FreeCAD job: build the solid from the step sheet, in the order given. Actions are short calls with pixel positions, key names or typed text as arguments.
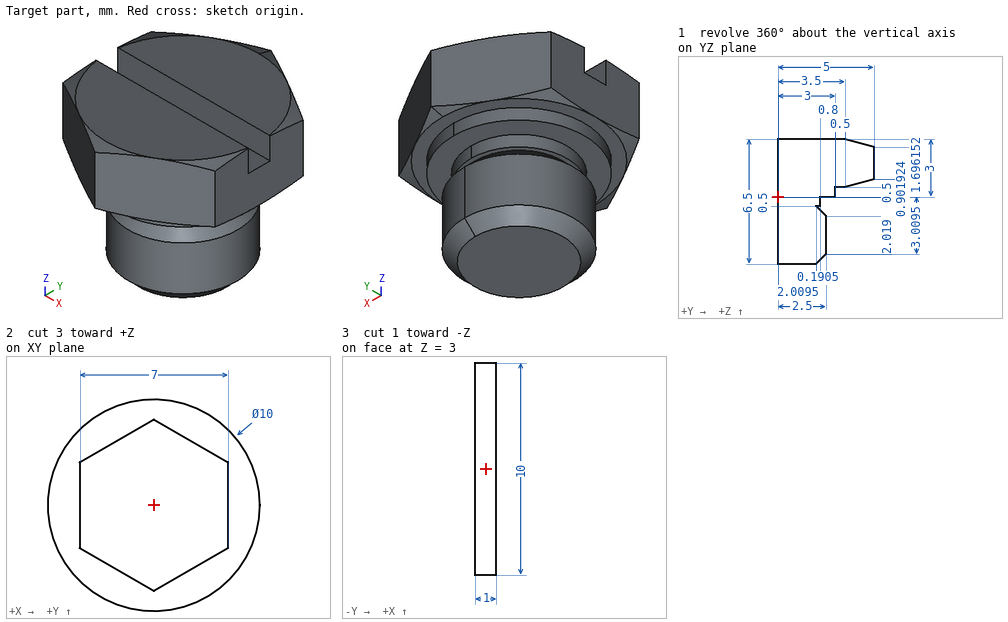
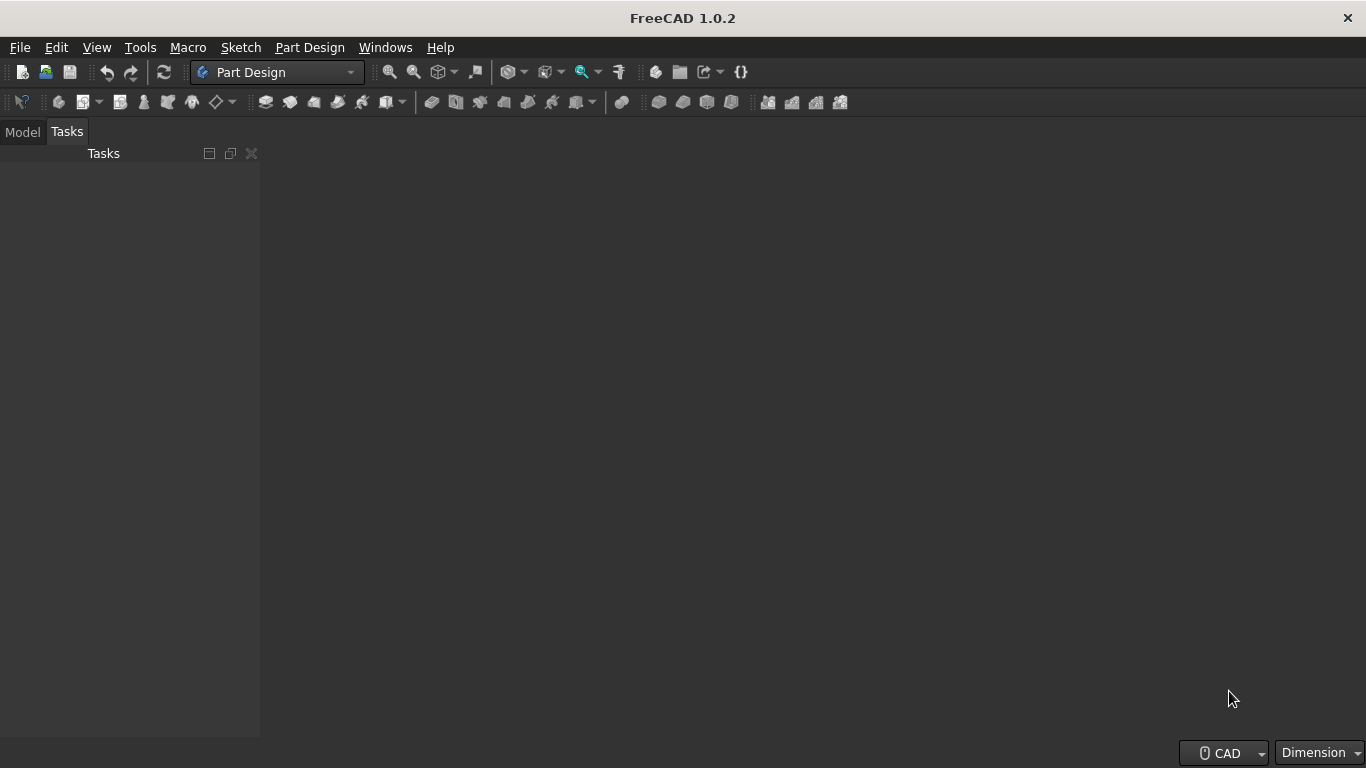
key(ctrl+n)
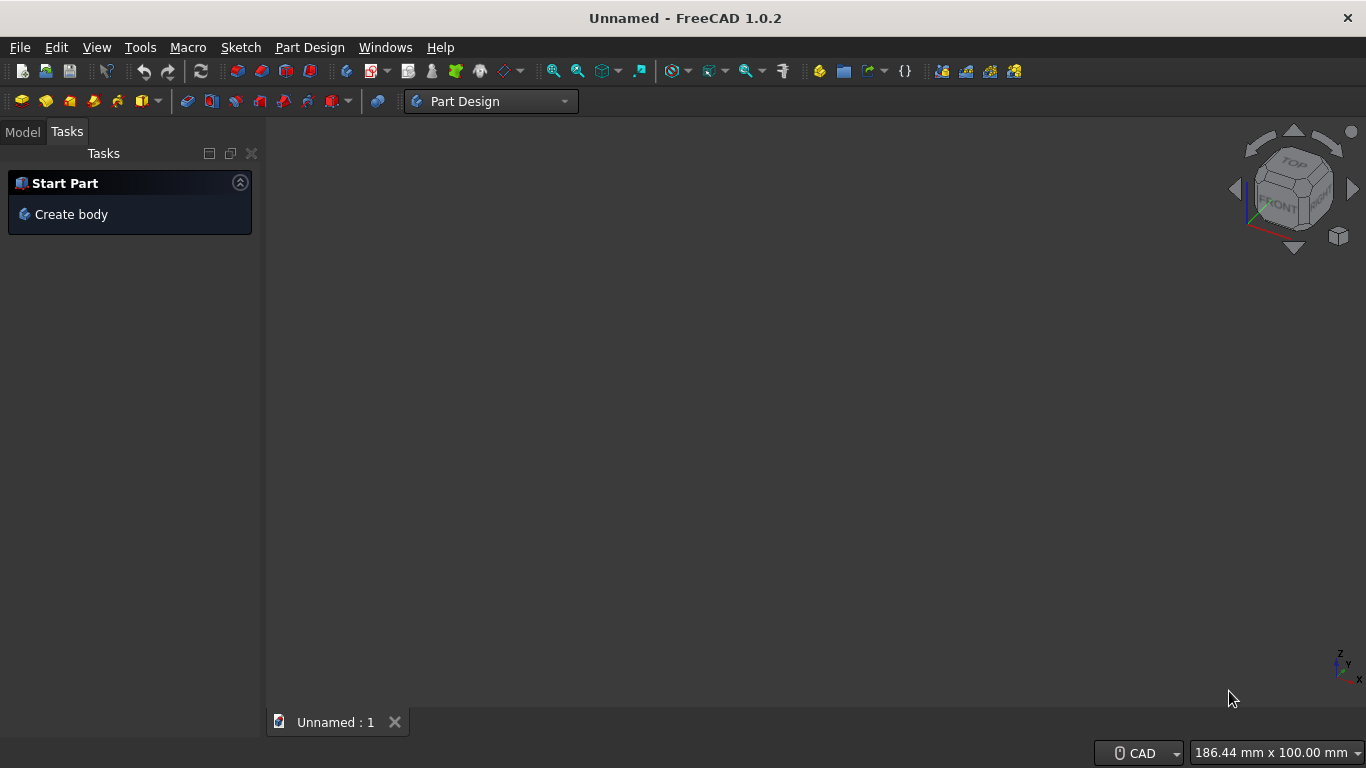
click(372, 72)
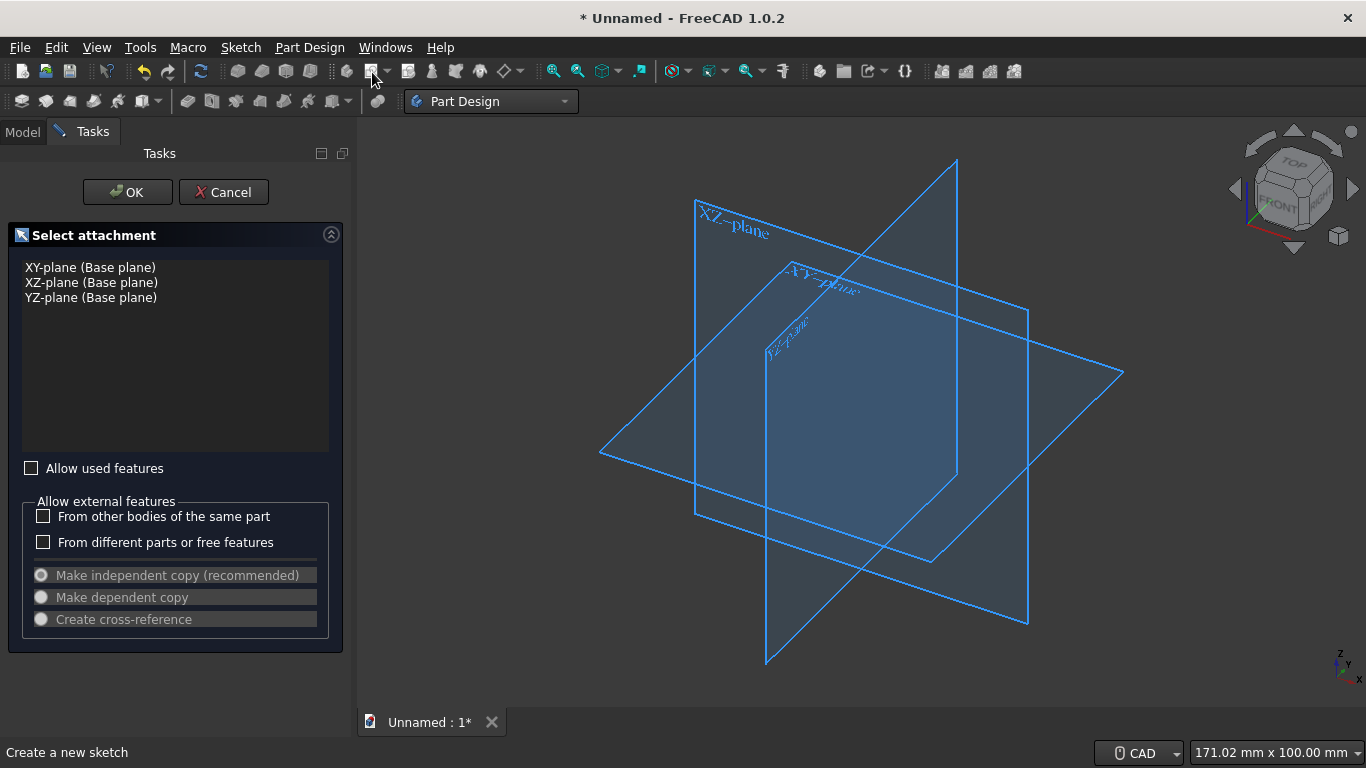
click(82, 298)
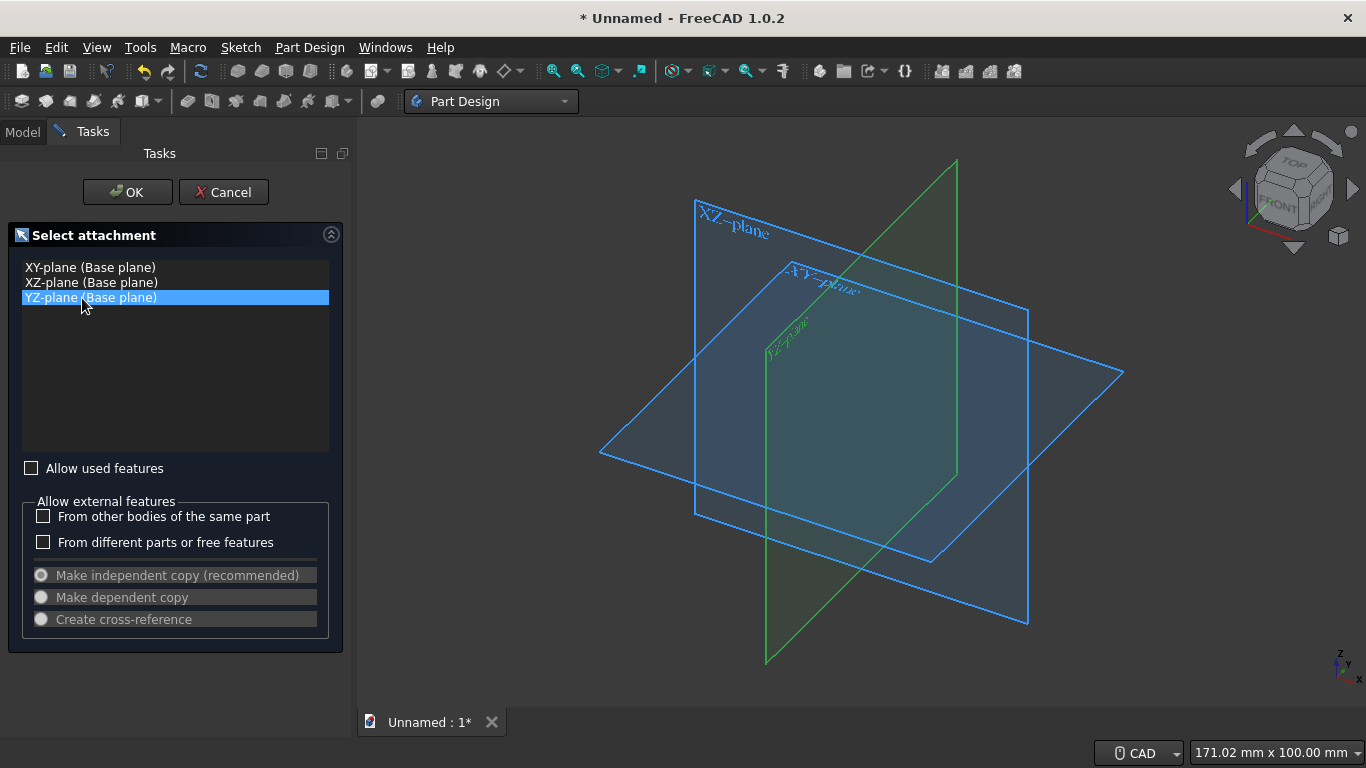
click(128, 192)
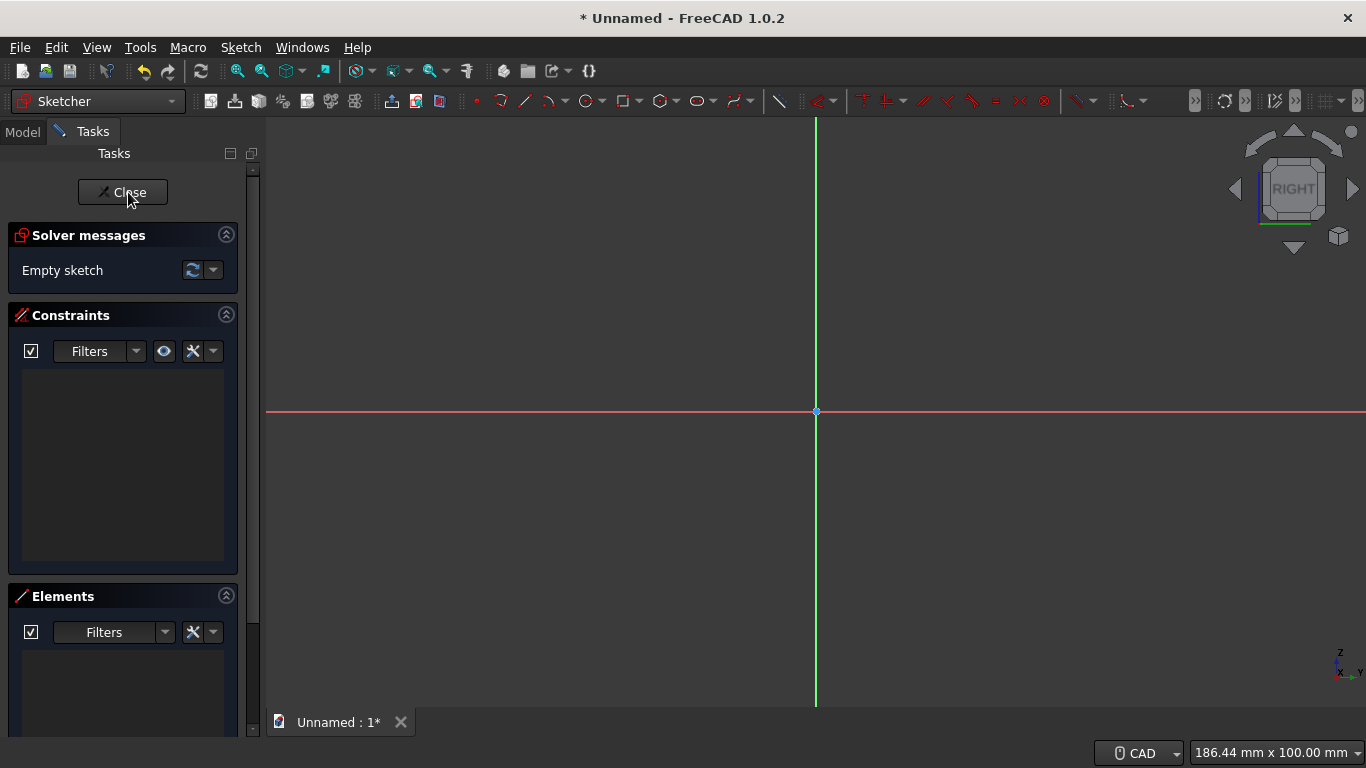
scroll(841, 414, up, 11)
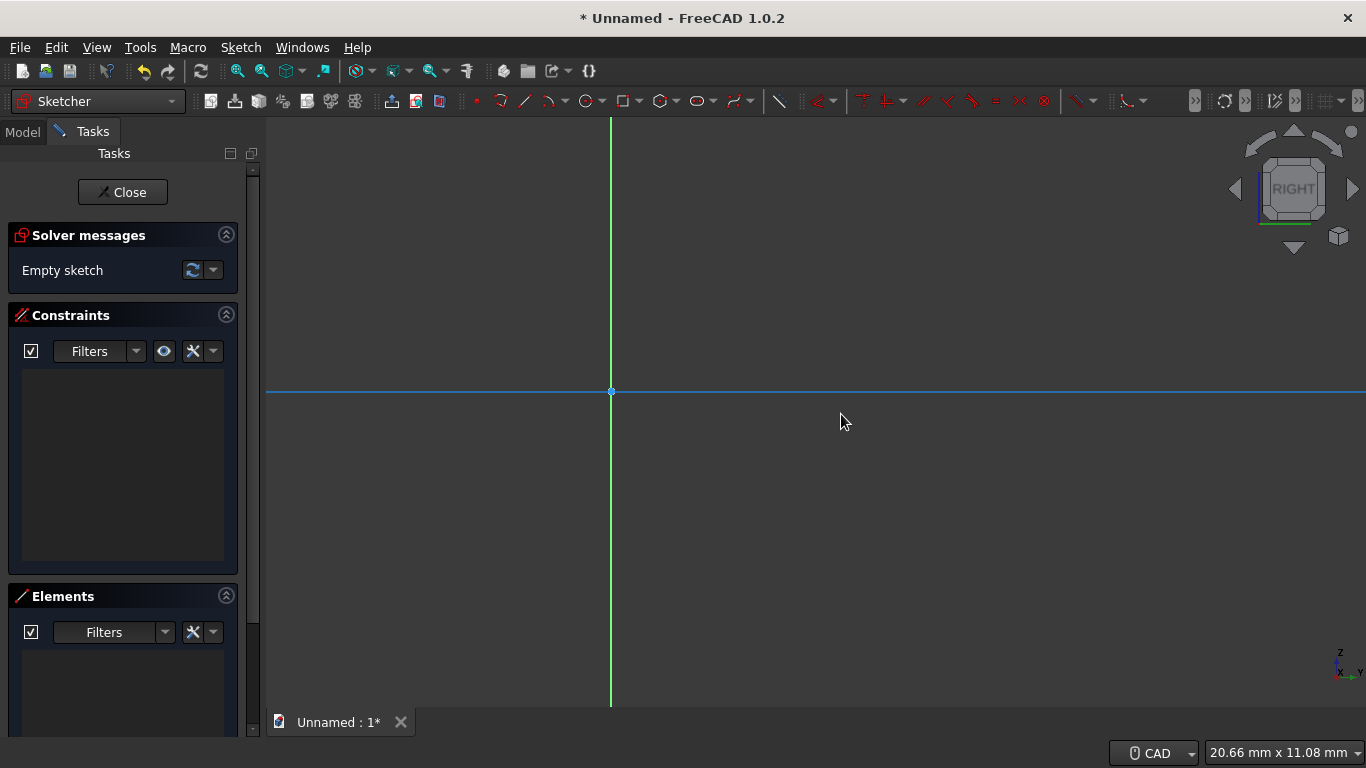
click(502, 102)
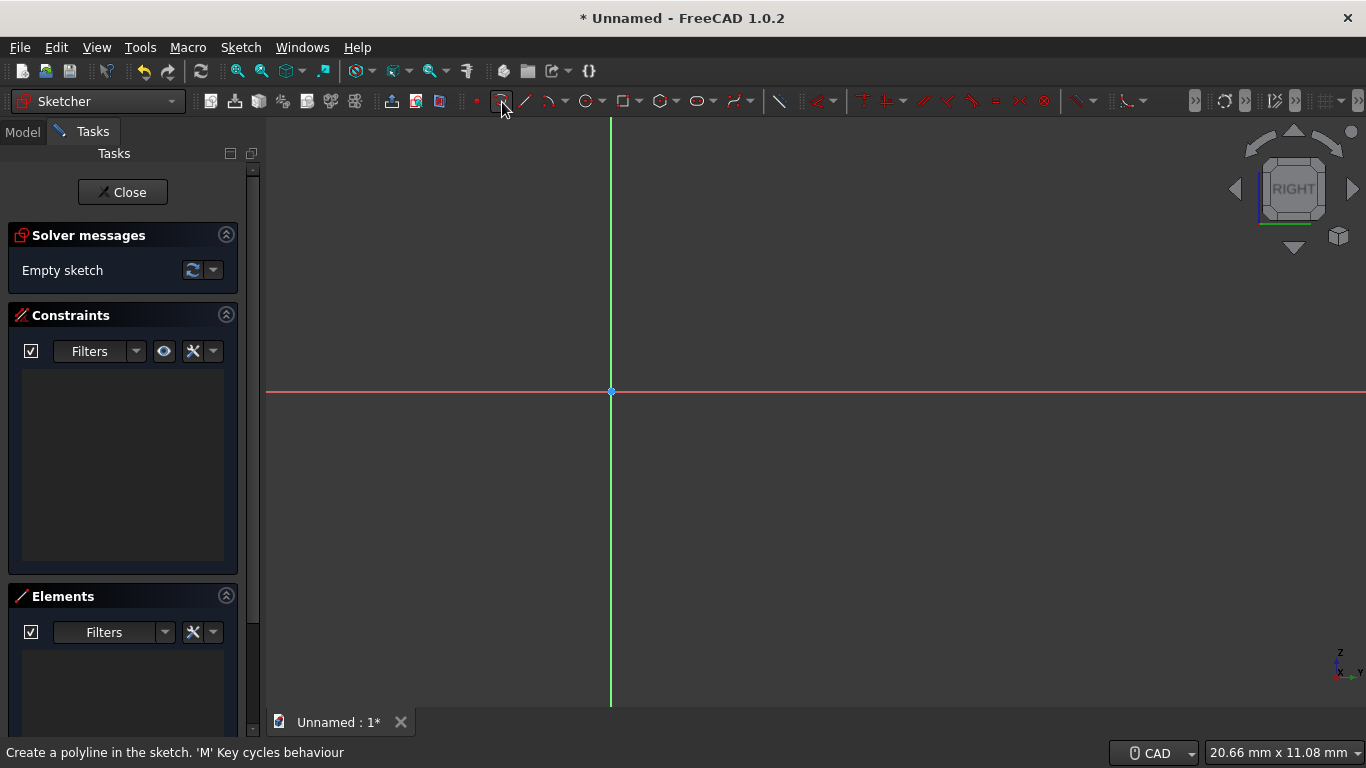
click(718, 419)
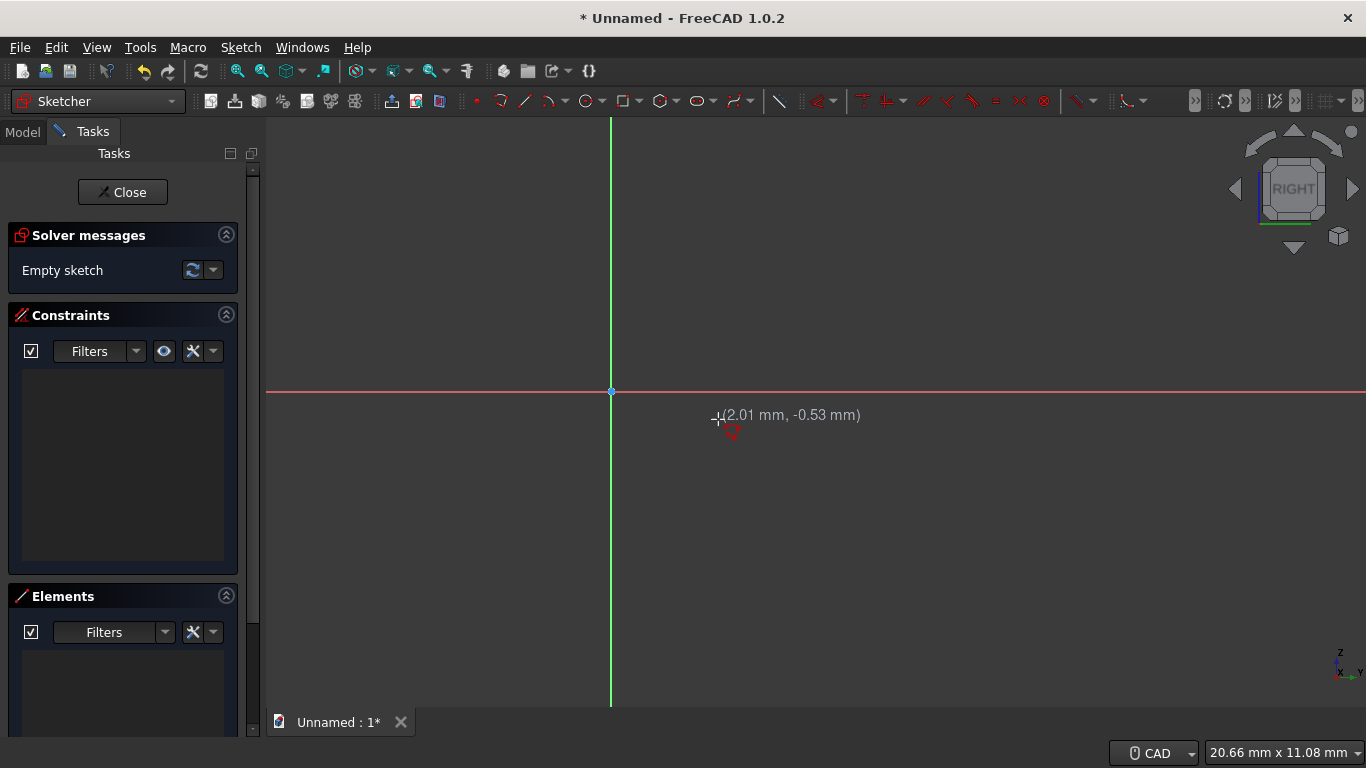
scroll(728, 419, up, 3)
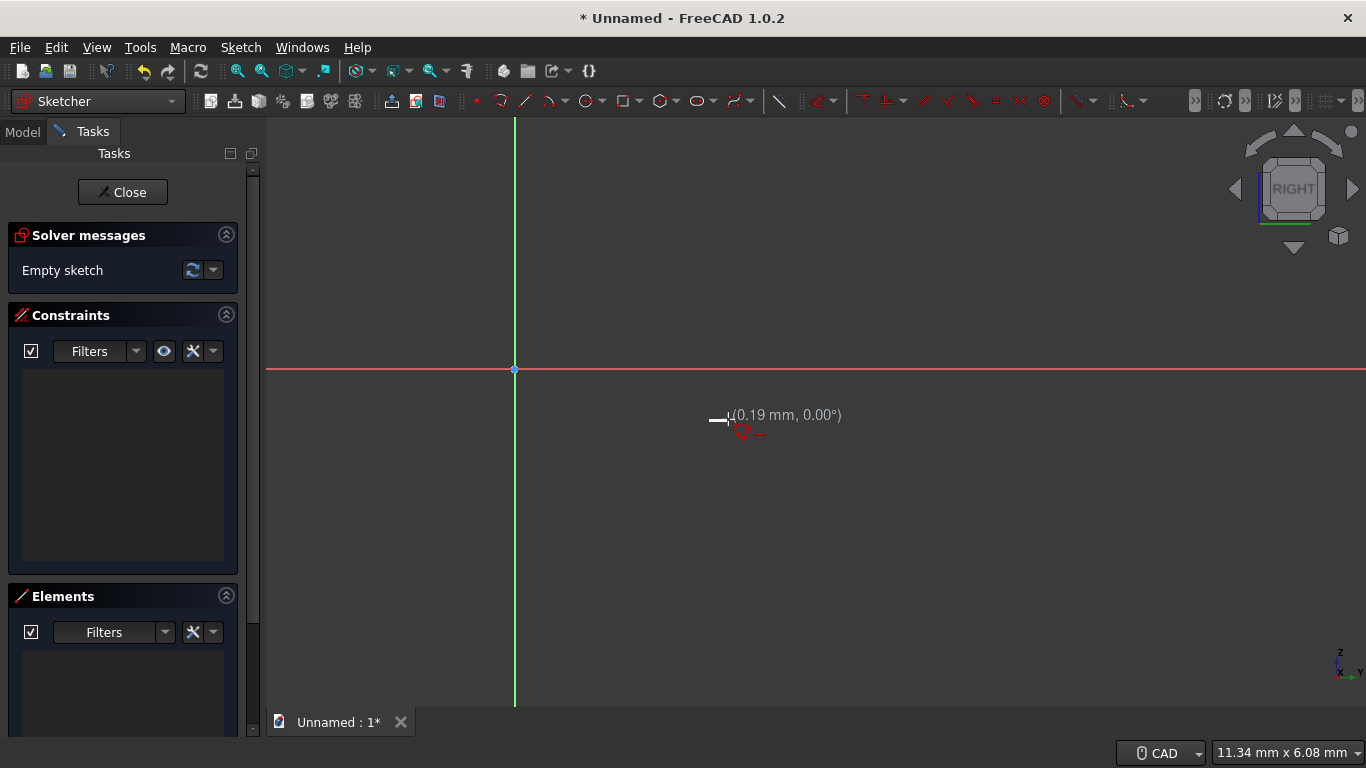
click(728, 419)
click(728, 369)
click(806, 378)
click(806, 321)
click(854, 321)
click(1000, 282)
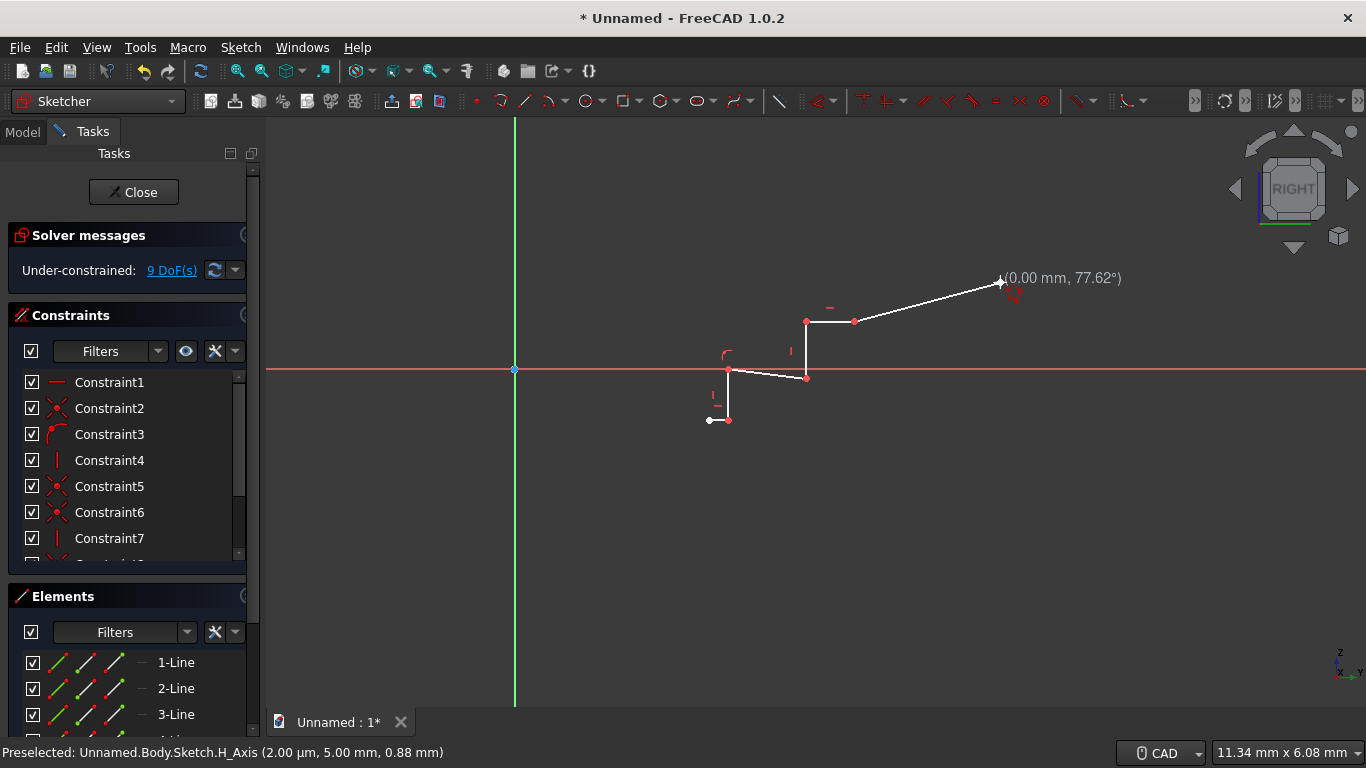
scroll(736, 435, down, 3)